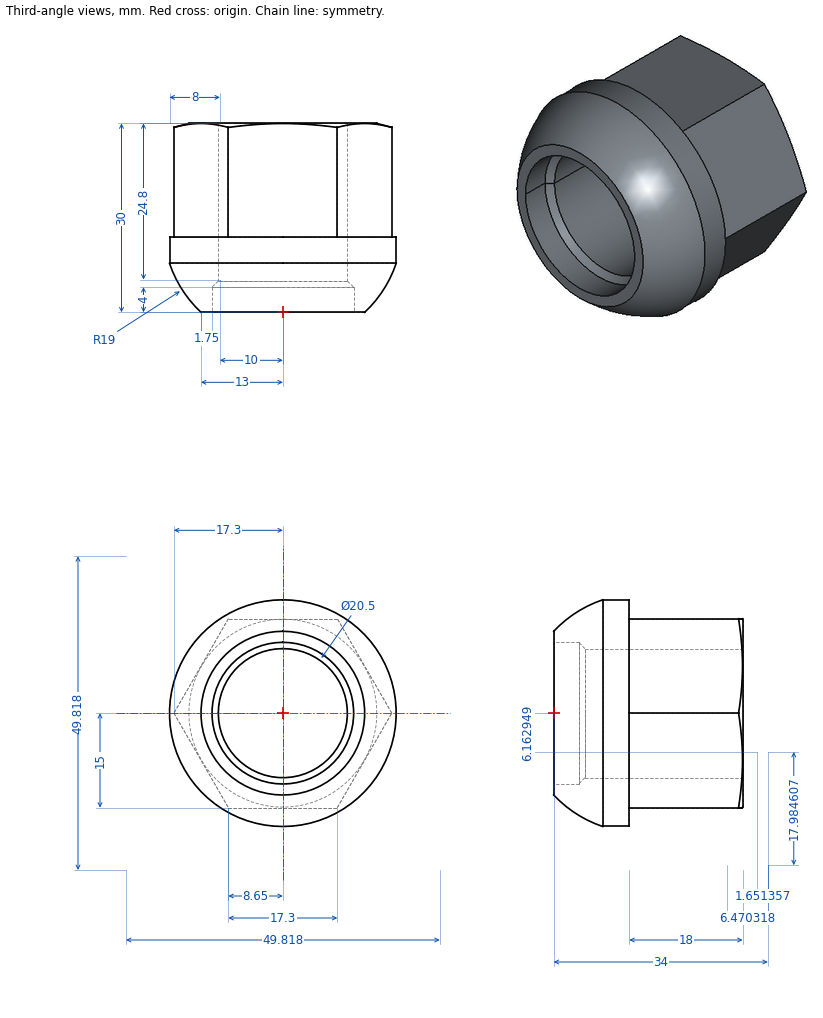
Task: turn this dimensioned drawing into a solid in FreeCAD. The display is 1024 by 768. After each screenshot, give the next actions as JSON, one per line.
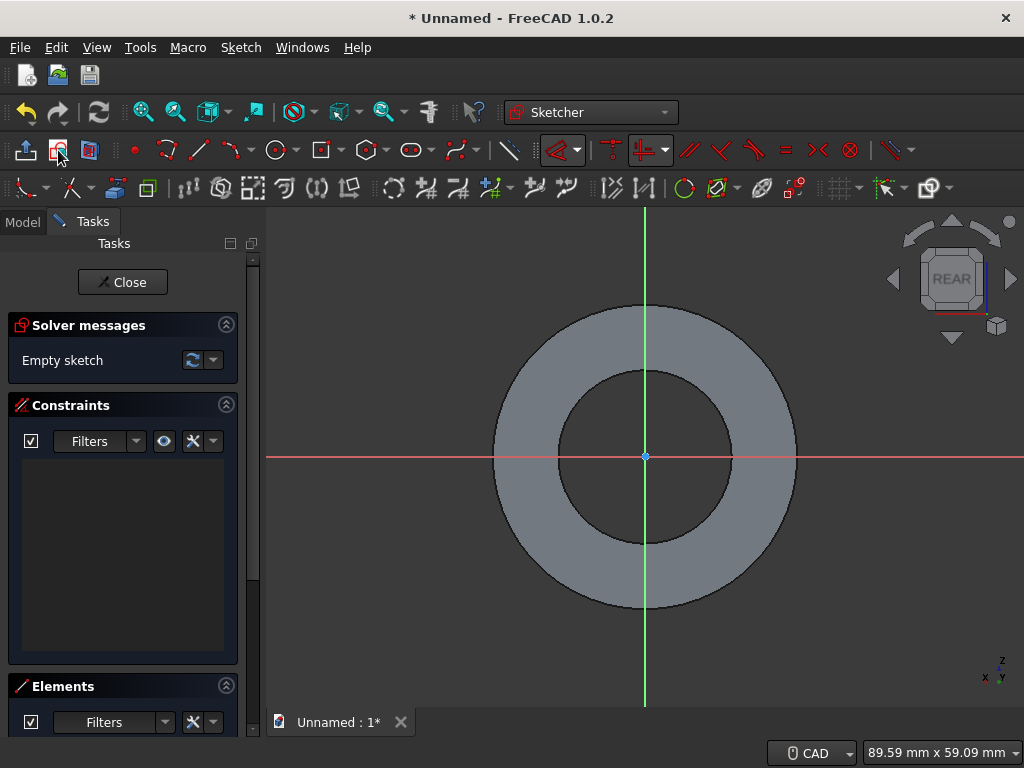
{"action": "scroll", "coordinate": [294, 457], "scroll_direction": "down", "scroll_amount": 1}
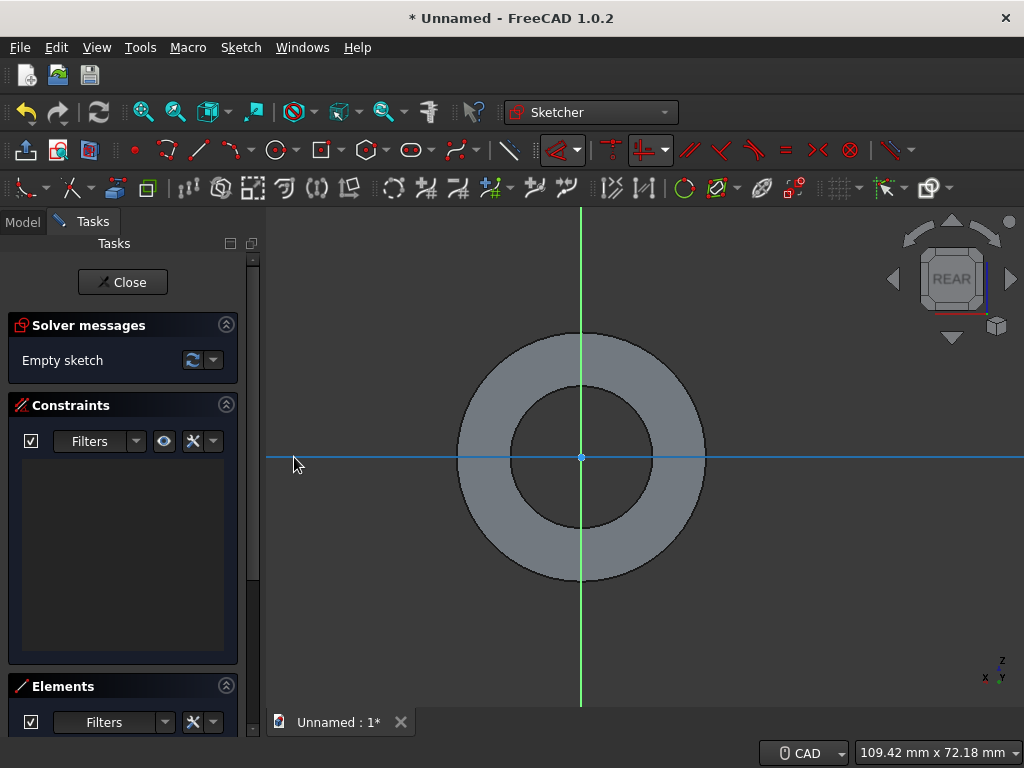
{"action": "key", "text": "g v"}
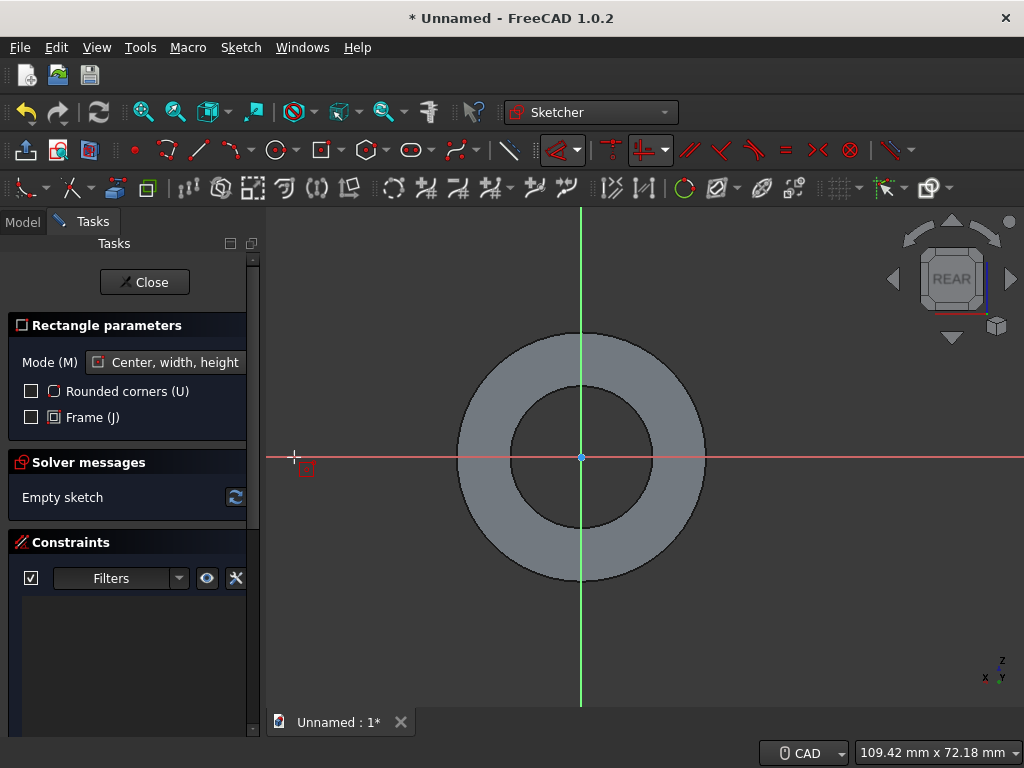
{"action": "left_click", "coordinate": [581, 457]}
{"action": "left_click", "coordinate": [754, 285]}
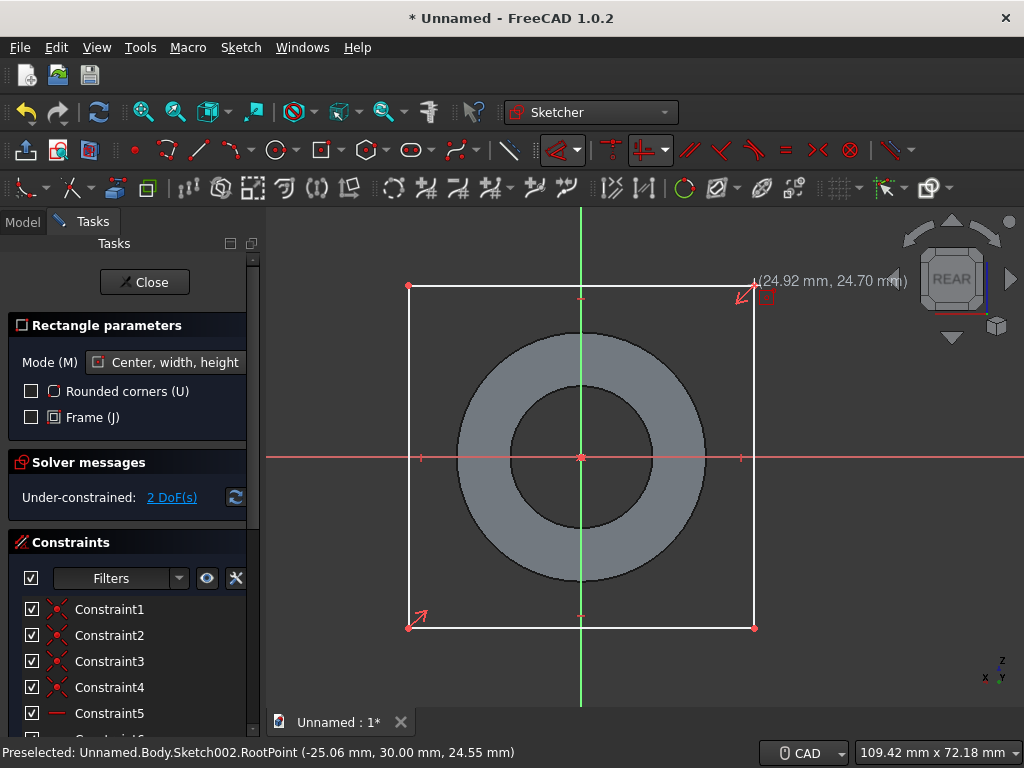
{"action": "key", "text": "g m"}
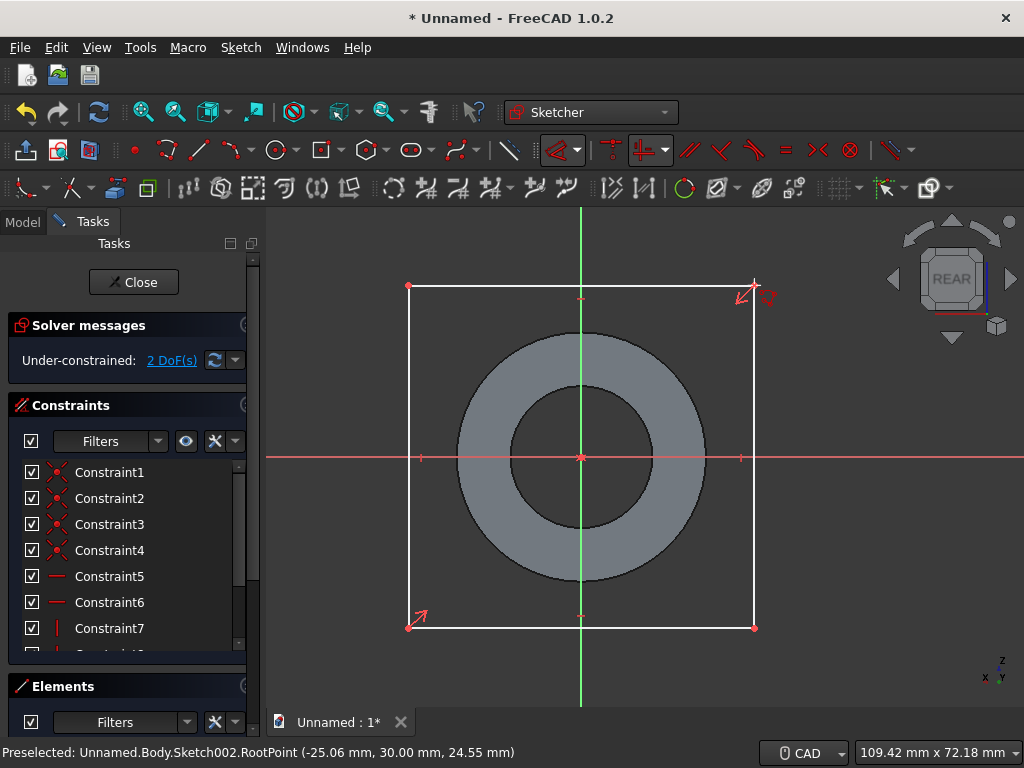
{"action": "left_click", "coordinate": [701, 457]}
{"action": "left_click", "coordinate": [641, 561]}
{"action": "left_click", "coordinate": [521, 561]}
{"action": "left_click", "coordinate": [462, 457]}
{"action": "left_click", "coordinate": [521, 353]}
{"action": "left_click", "coordinate": [641, 353]}
{"action": "left_click", "coordinate": [701, 457]}
{"action": "key", "text": "Escape"}
{"action": "key", "text": "Escape"}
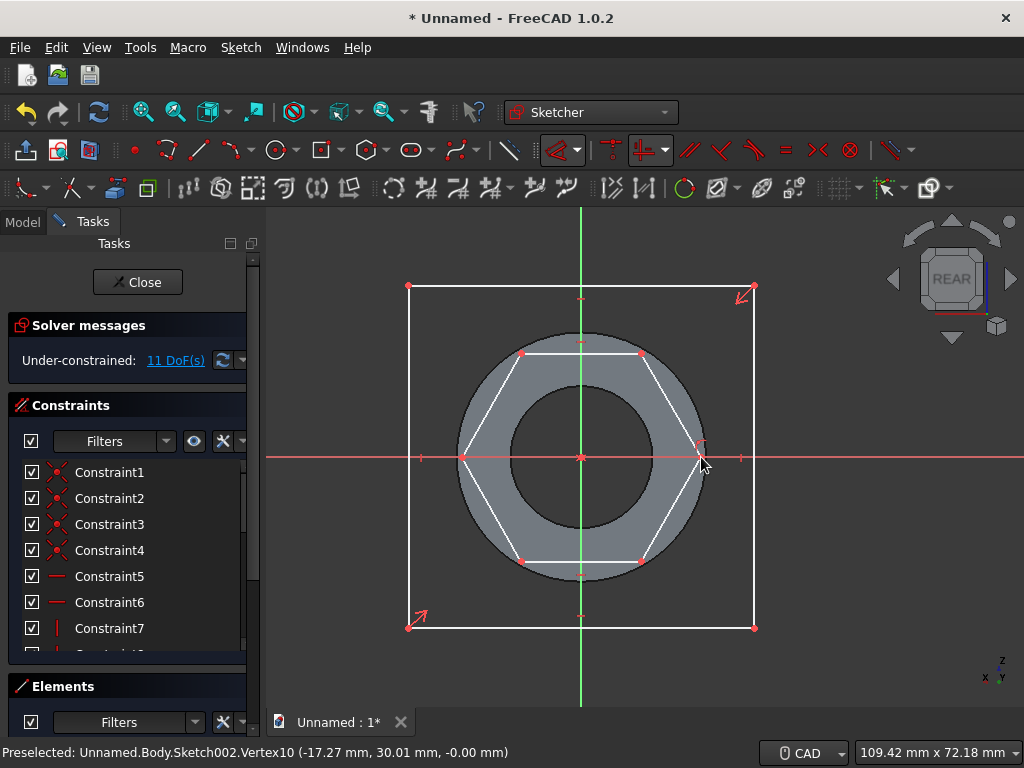
{"action": "left_click", "coordinate": [701, 457]}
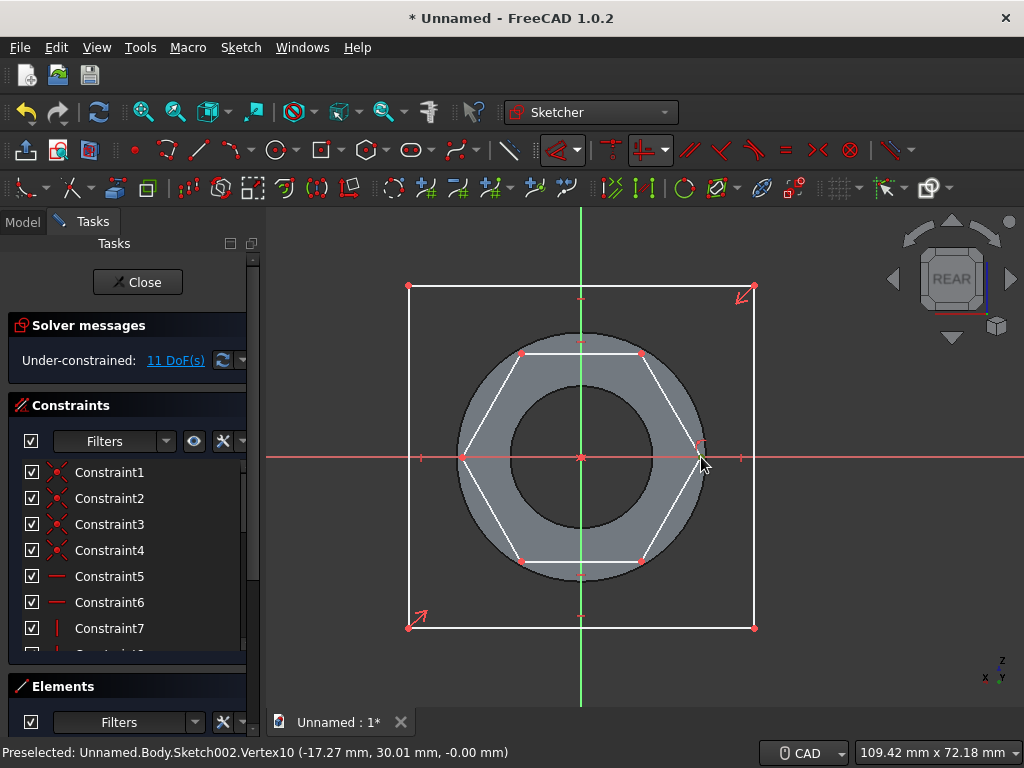
{"action": "left_click", "coordinate": [462, 458]}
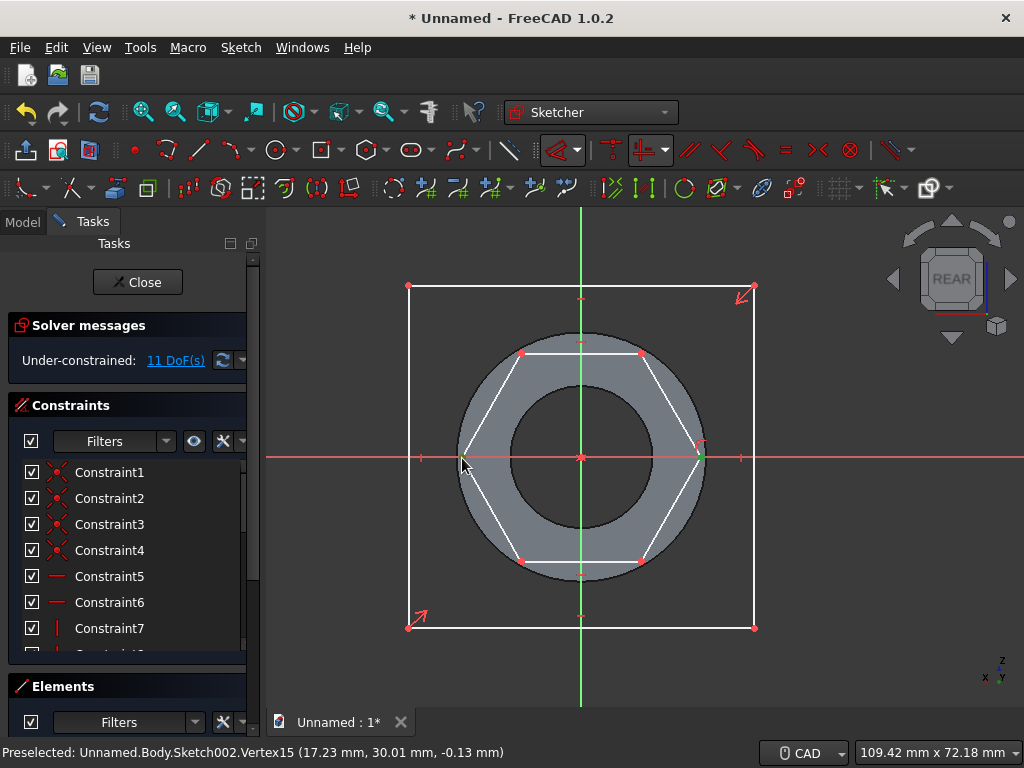
{"action": "left_click", "coordinate": [581, 520]}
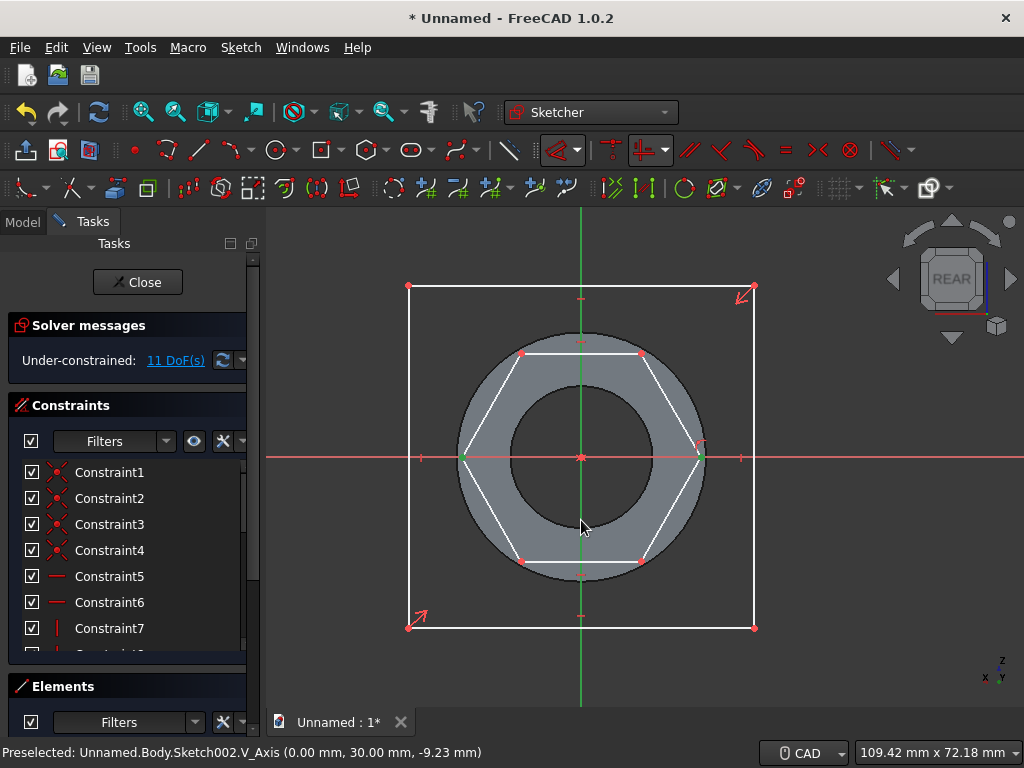
{"action": "left_click", "coordinate": [818, 150]}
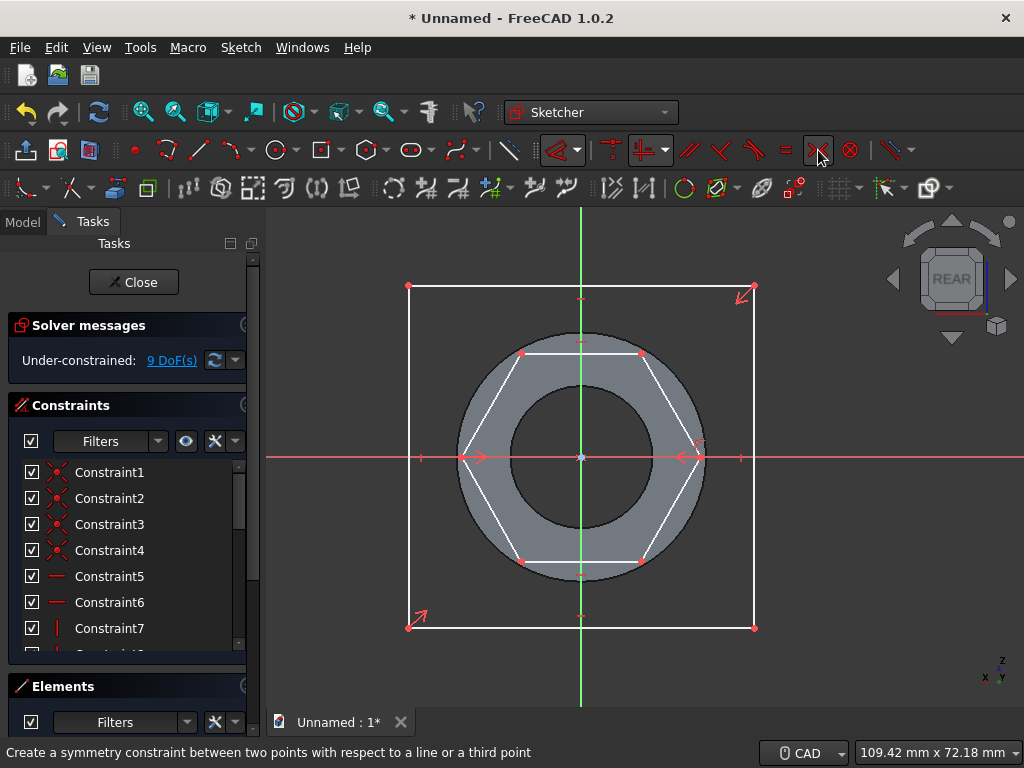
{"action": "left_click", "coordinate": [521, 562]}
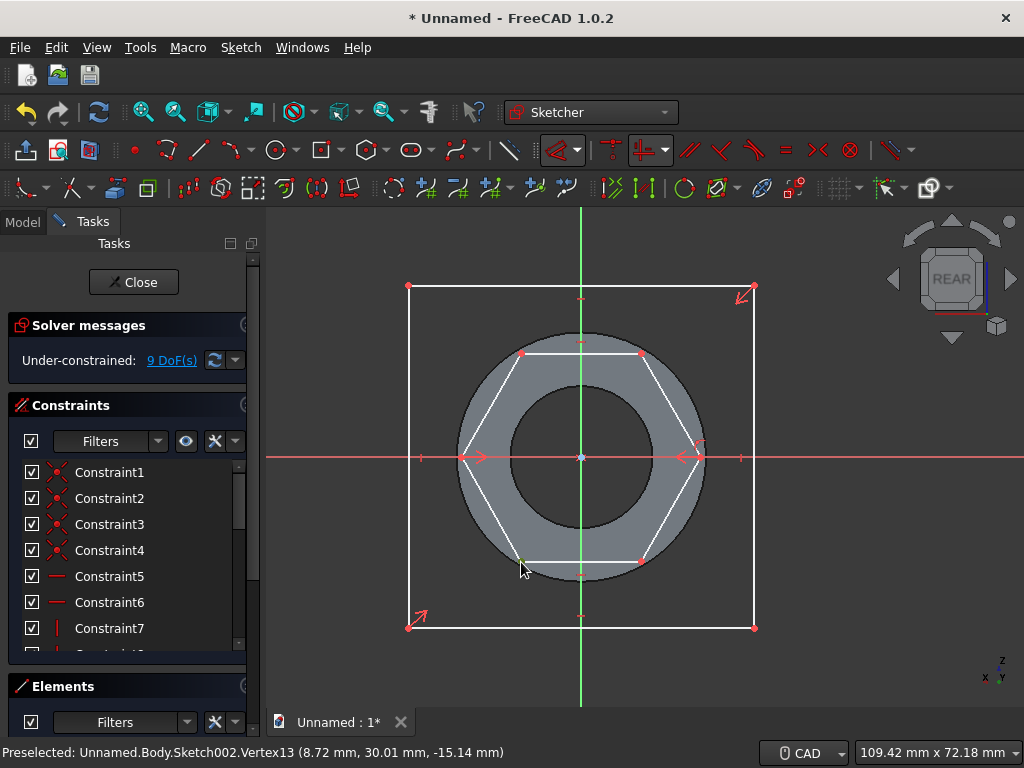
{"action": "left_click", "coordinate": [521, 354]}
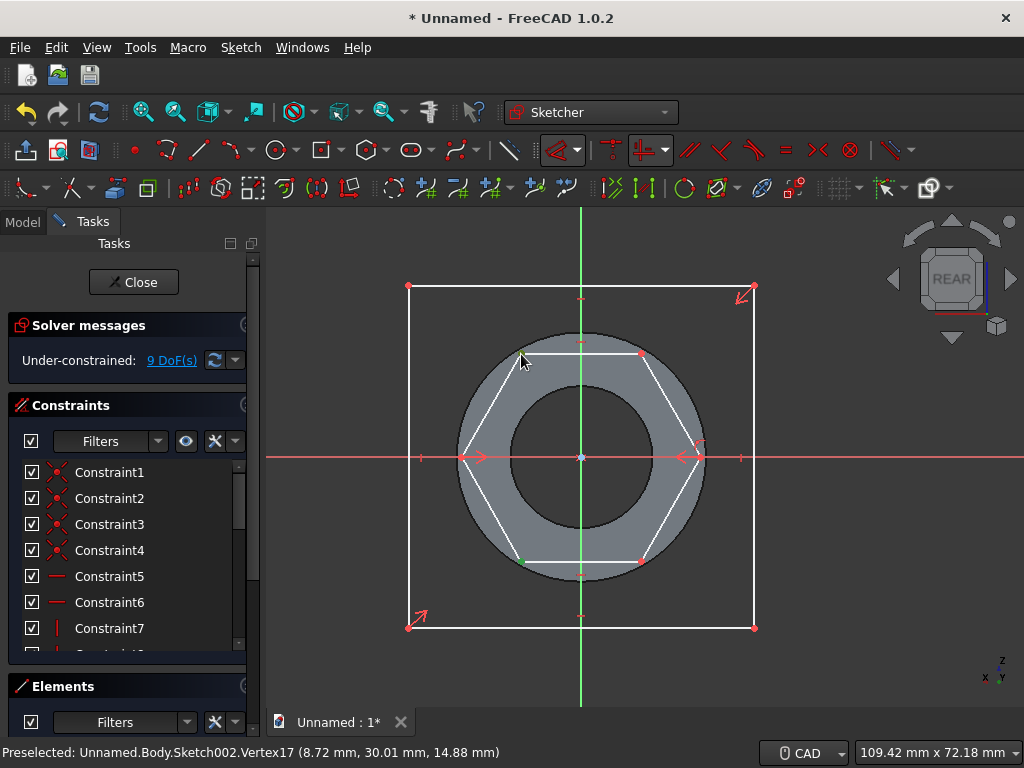
{"action": "left_click", "coordinate": [334, 457]}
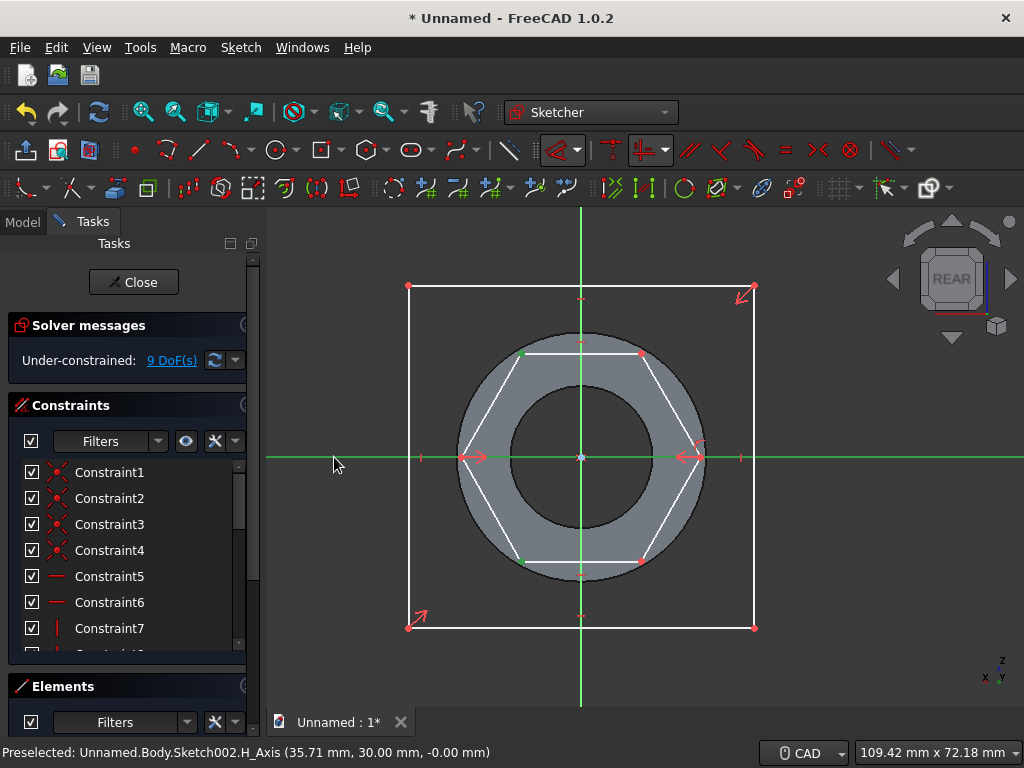
{"action": "key", "text": "s"}